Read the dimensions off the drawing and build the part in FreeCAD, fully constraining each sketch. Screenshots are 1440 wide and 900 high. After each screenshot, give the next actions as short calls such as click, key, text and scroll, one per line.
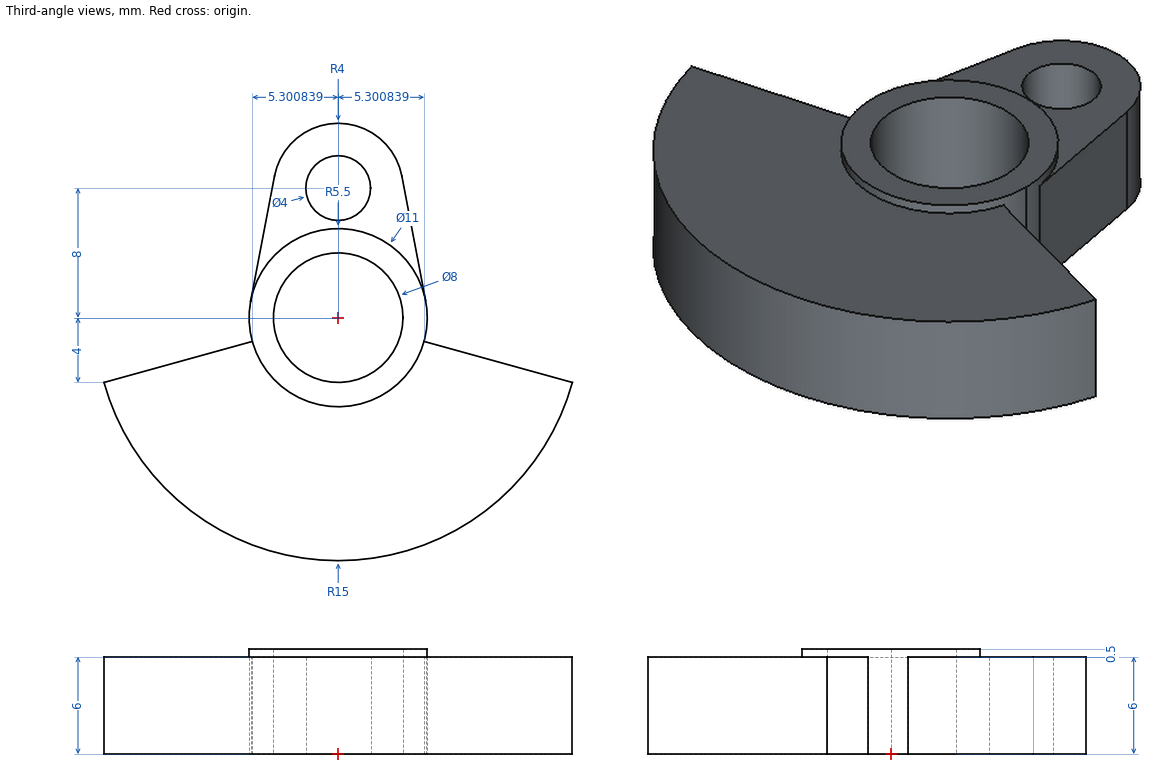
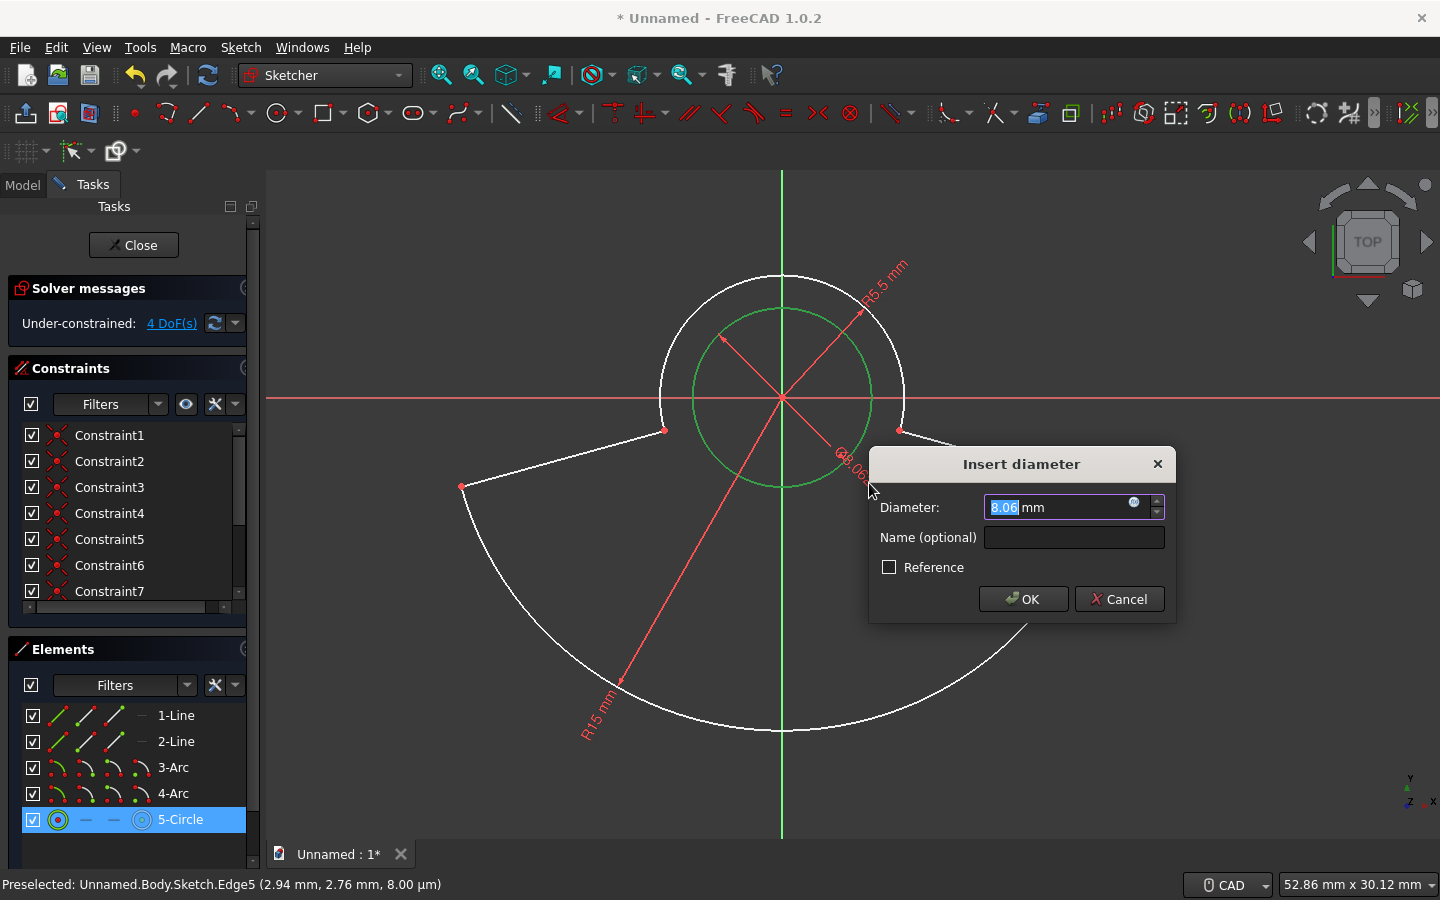
text(8)
key(Return)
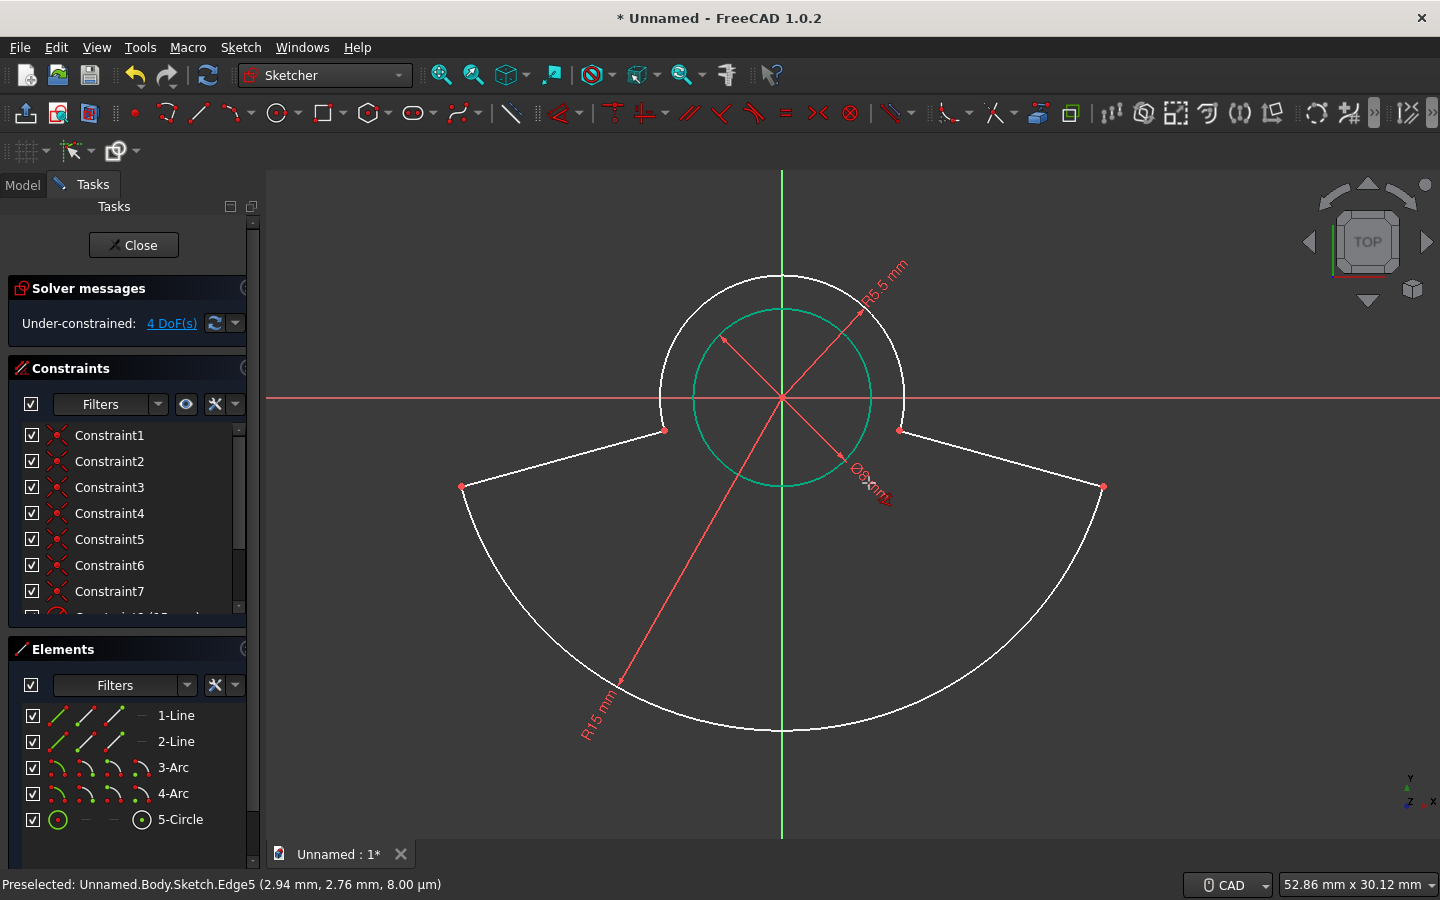
click(461, 487)
click(427, 442)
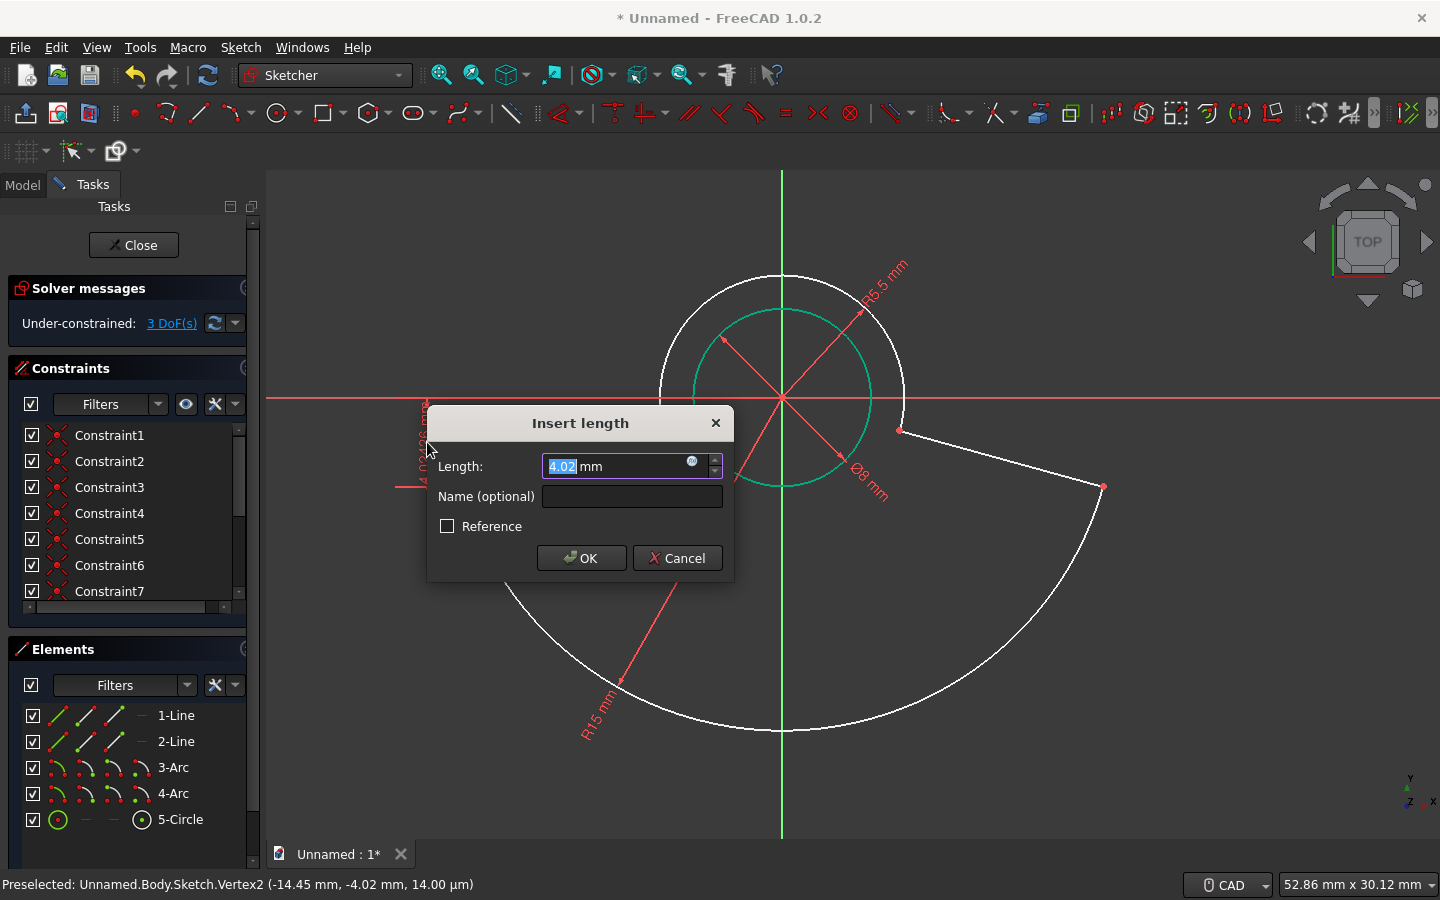
text(4)
key(Return)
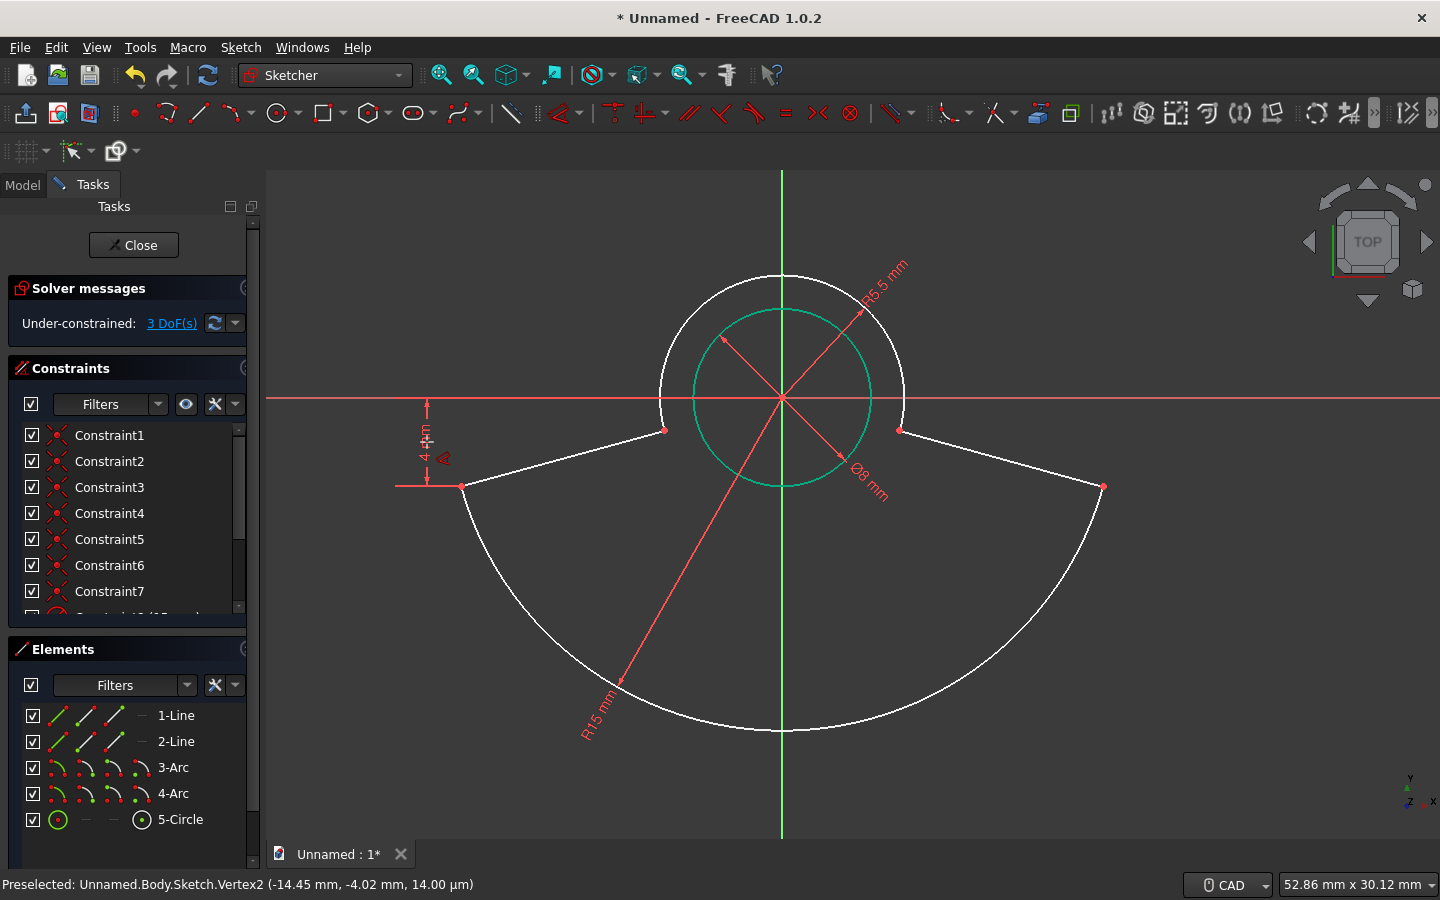
click(1103, 487)
click(1137, 442)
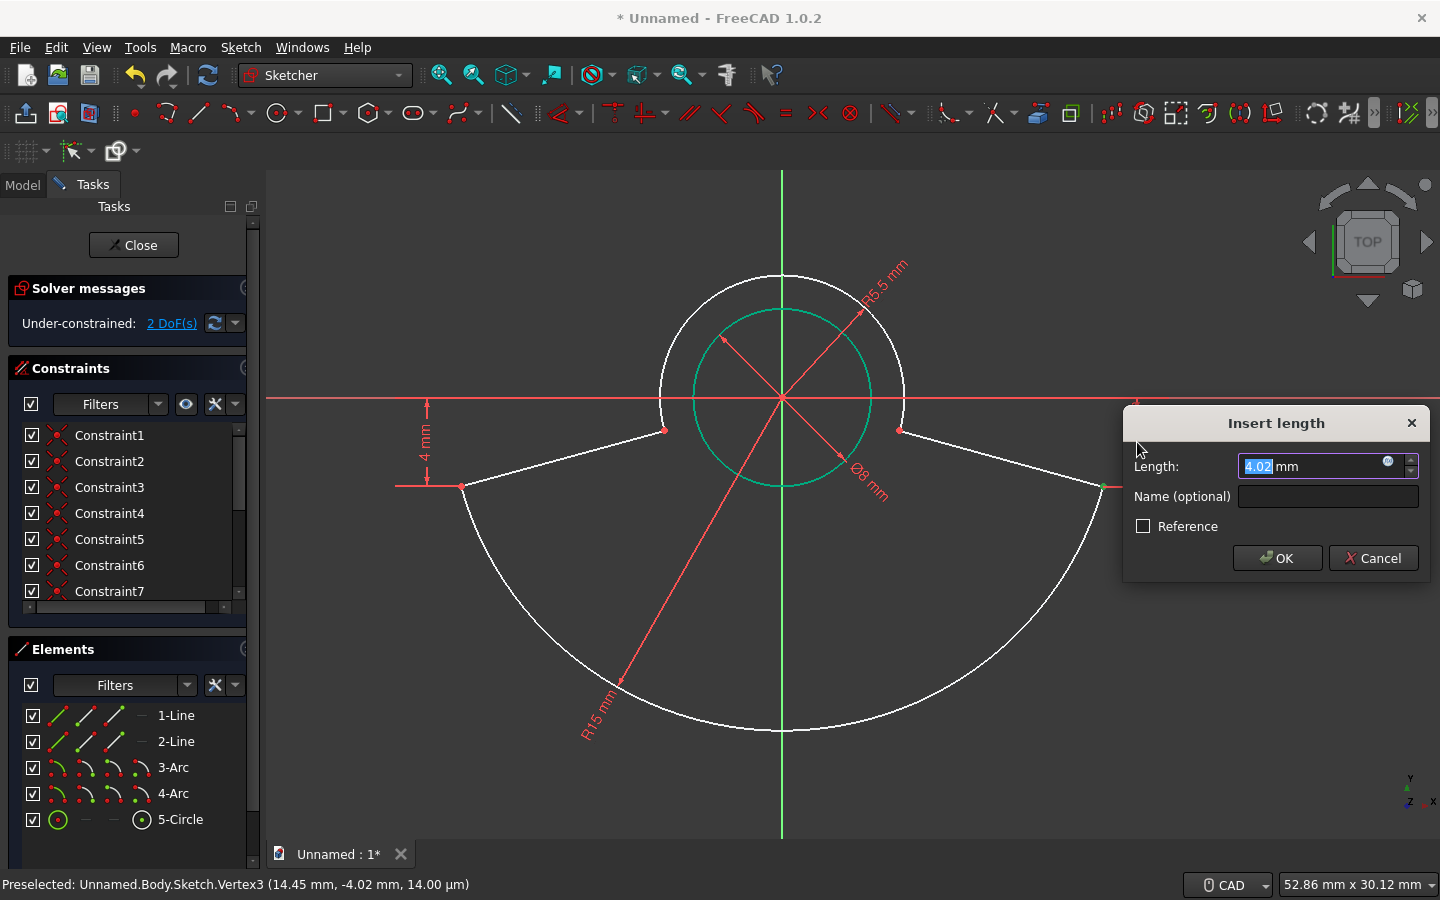
text(4)
key(Return)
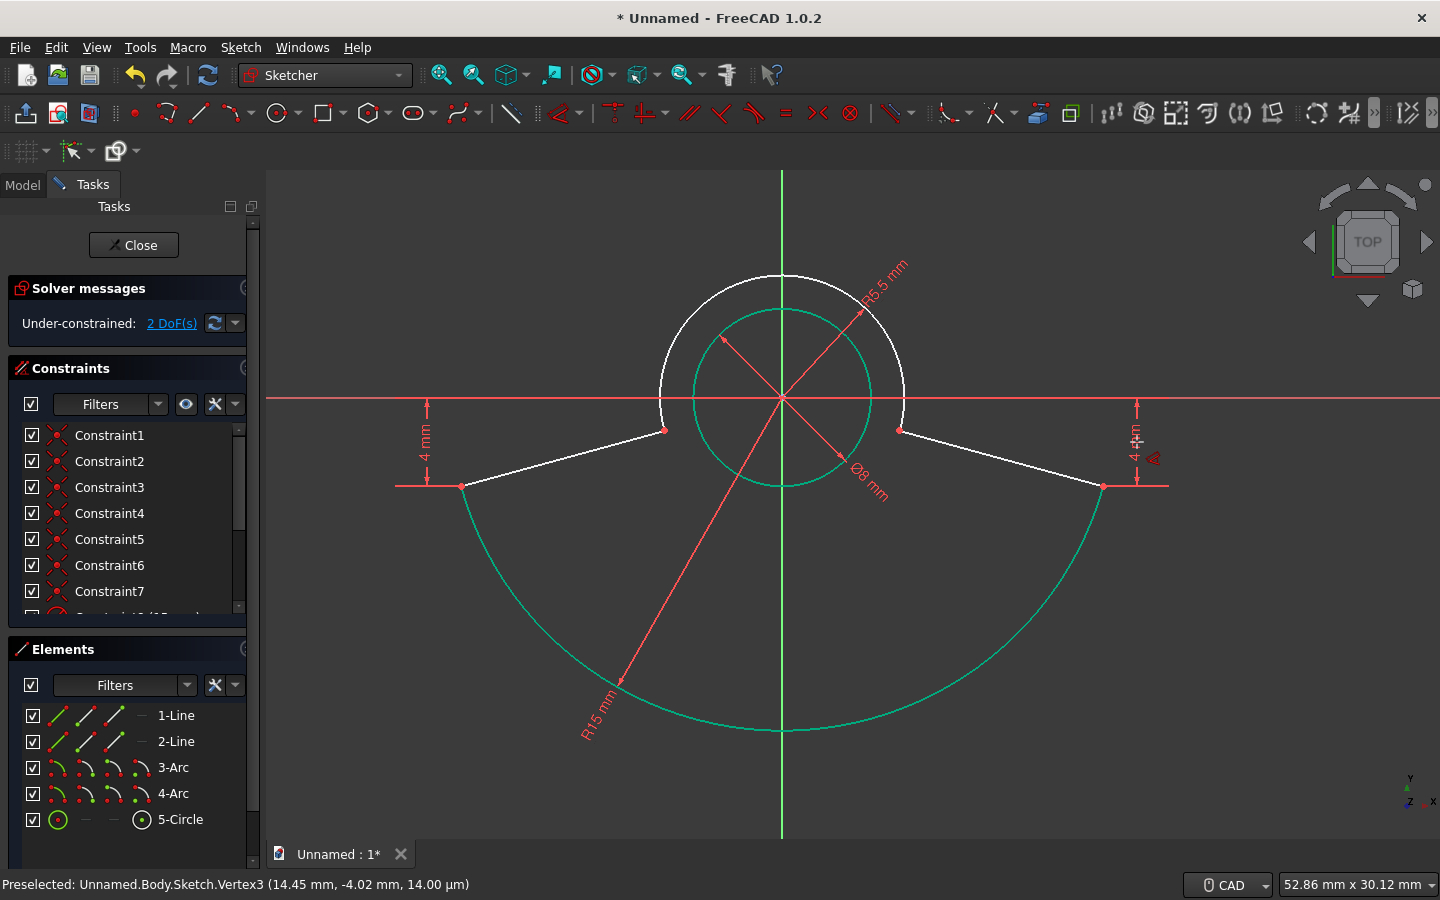
click(665, 431)
click(723, 364)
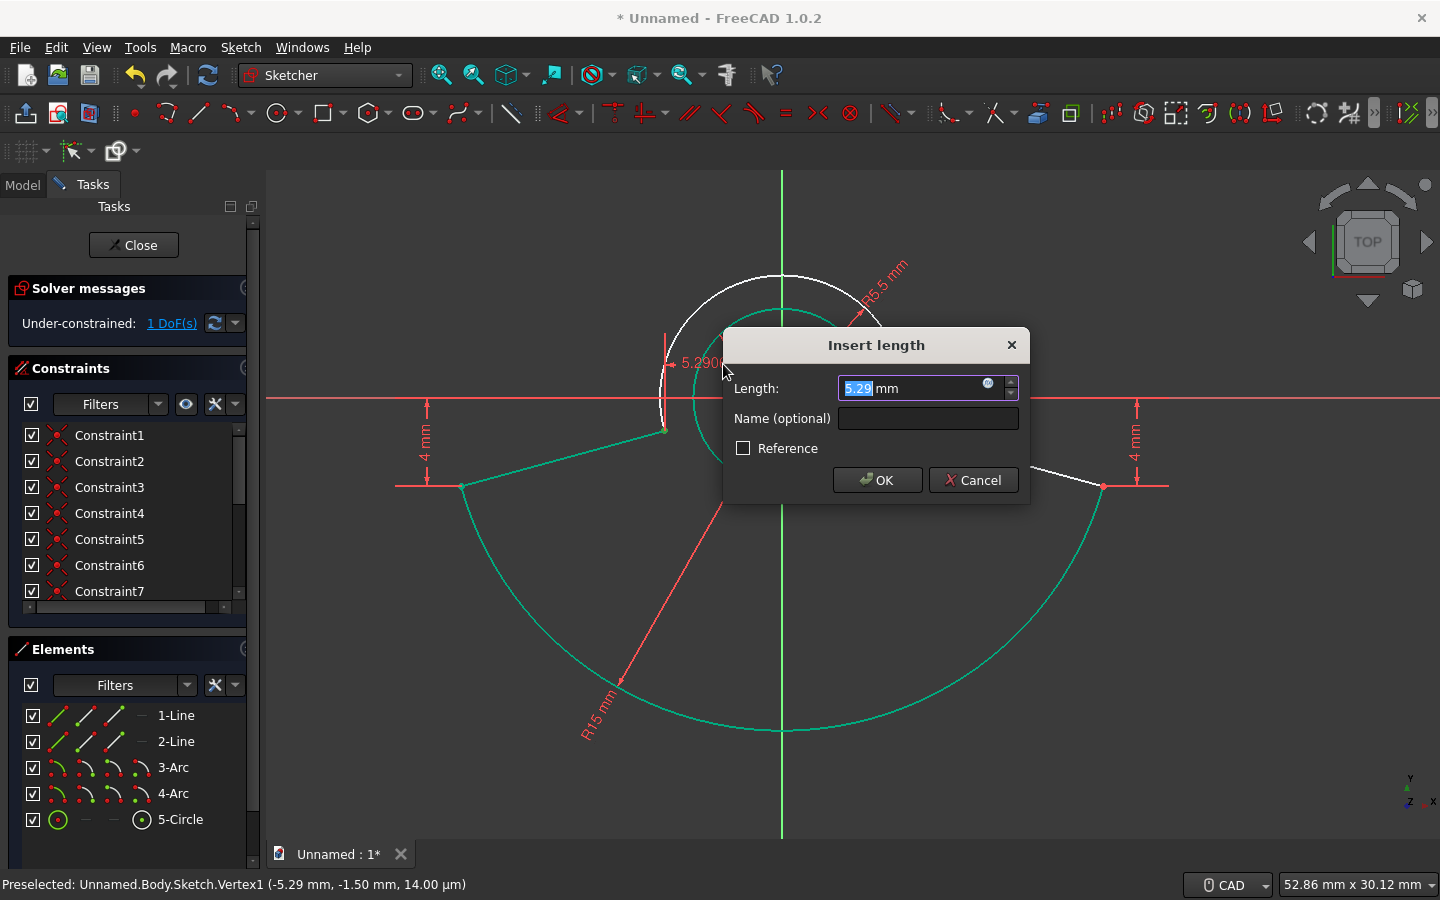
text(5.300839)
key(Return)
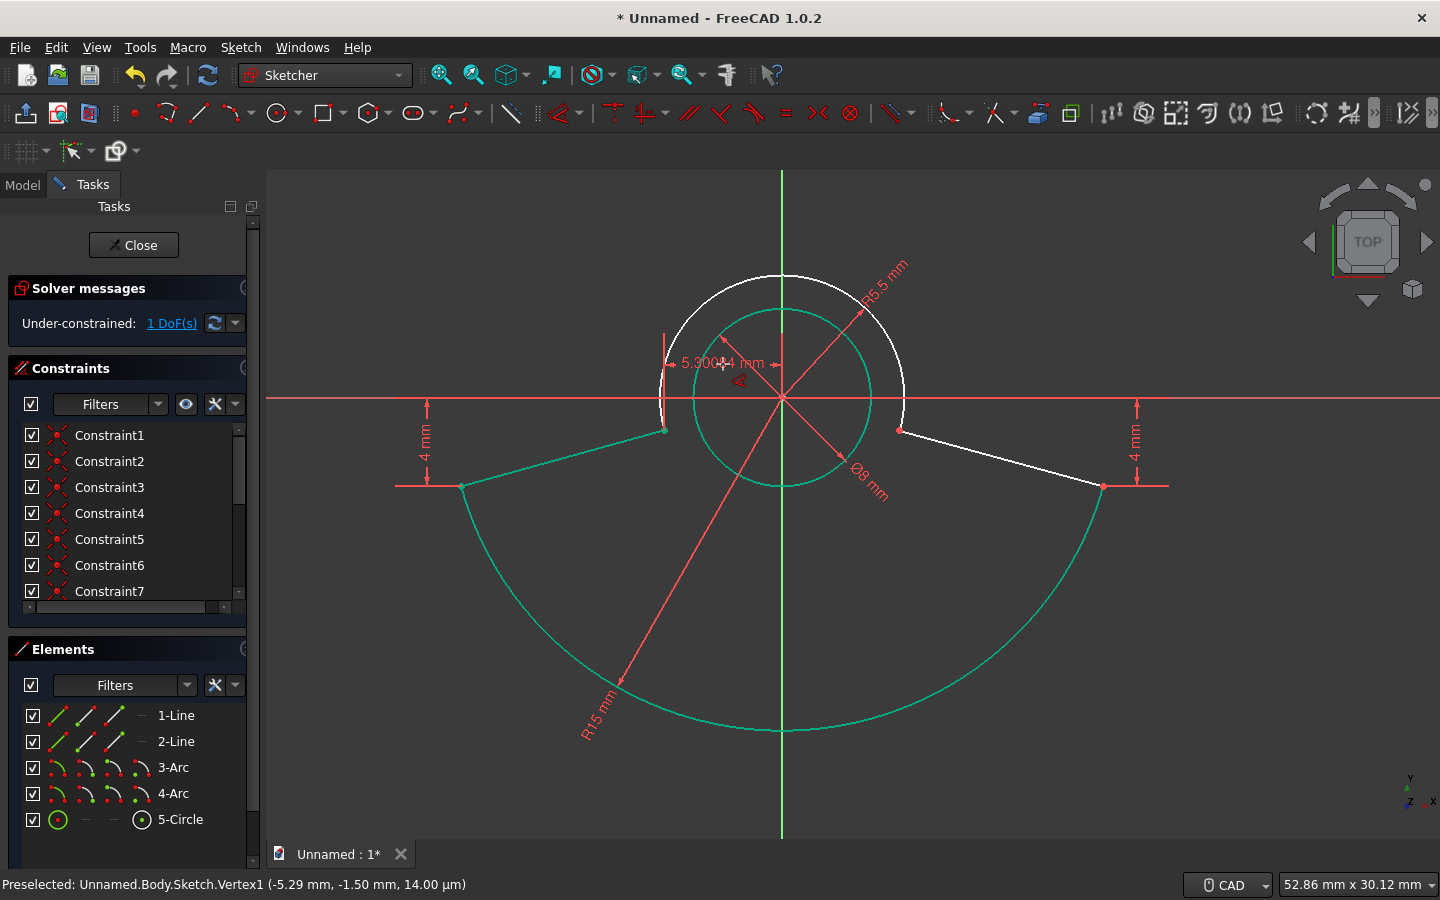
click(900, 431)
click(841, 364)